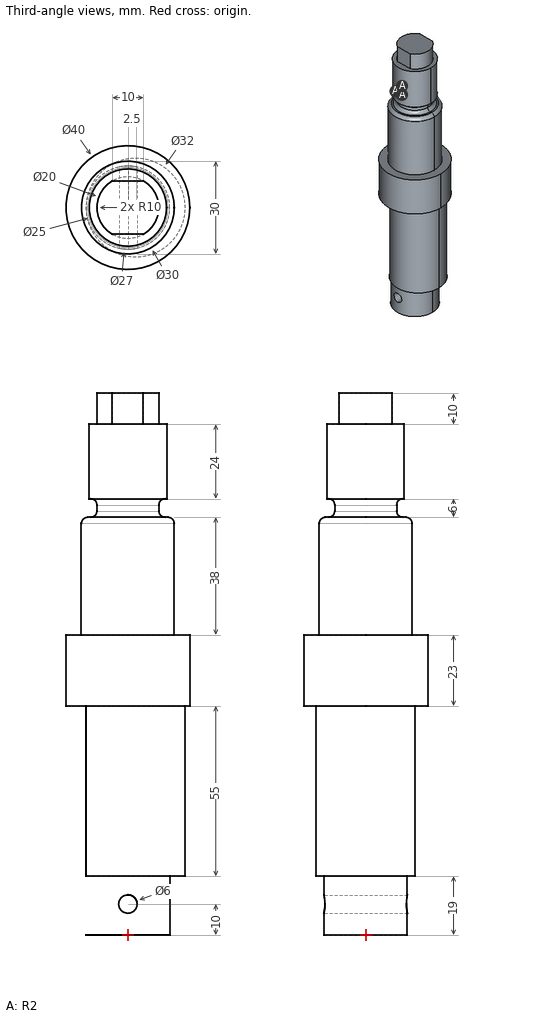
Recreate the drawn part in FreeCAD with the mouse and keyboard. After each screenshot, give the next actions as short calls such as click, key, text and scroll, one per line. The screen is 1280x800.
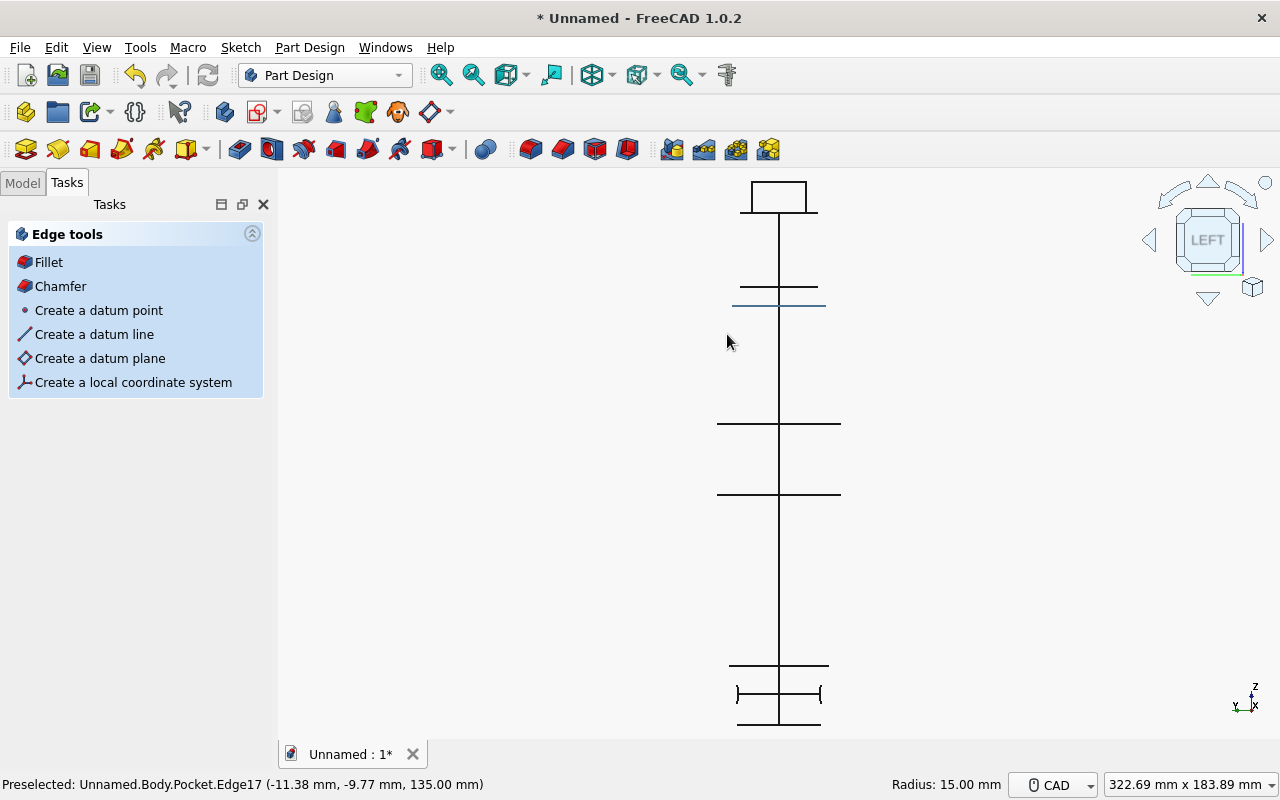
key(0)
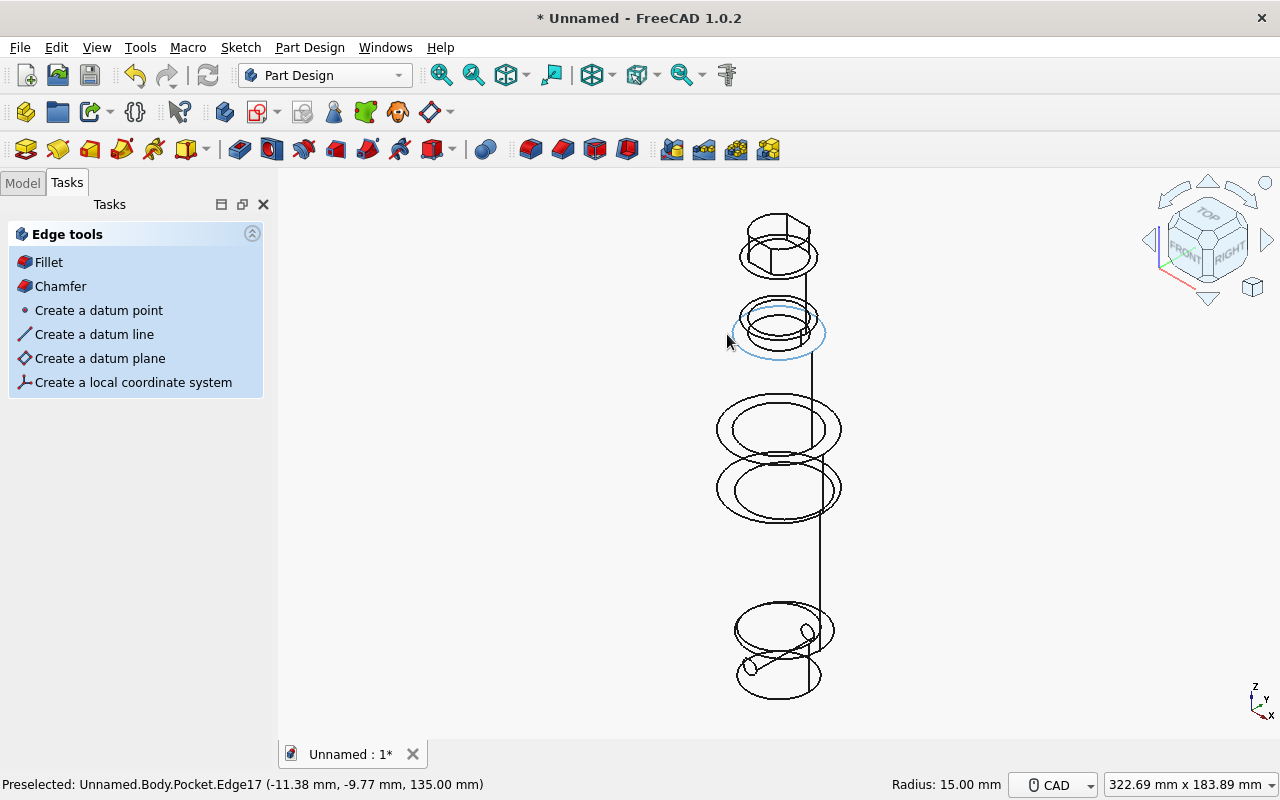
click(757, 319, ctrl)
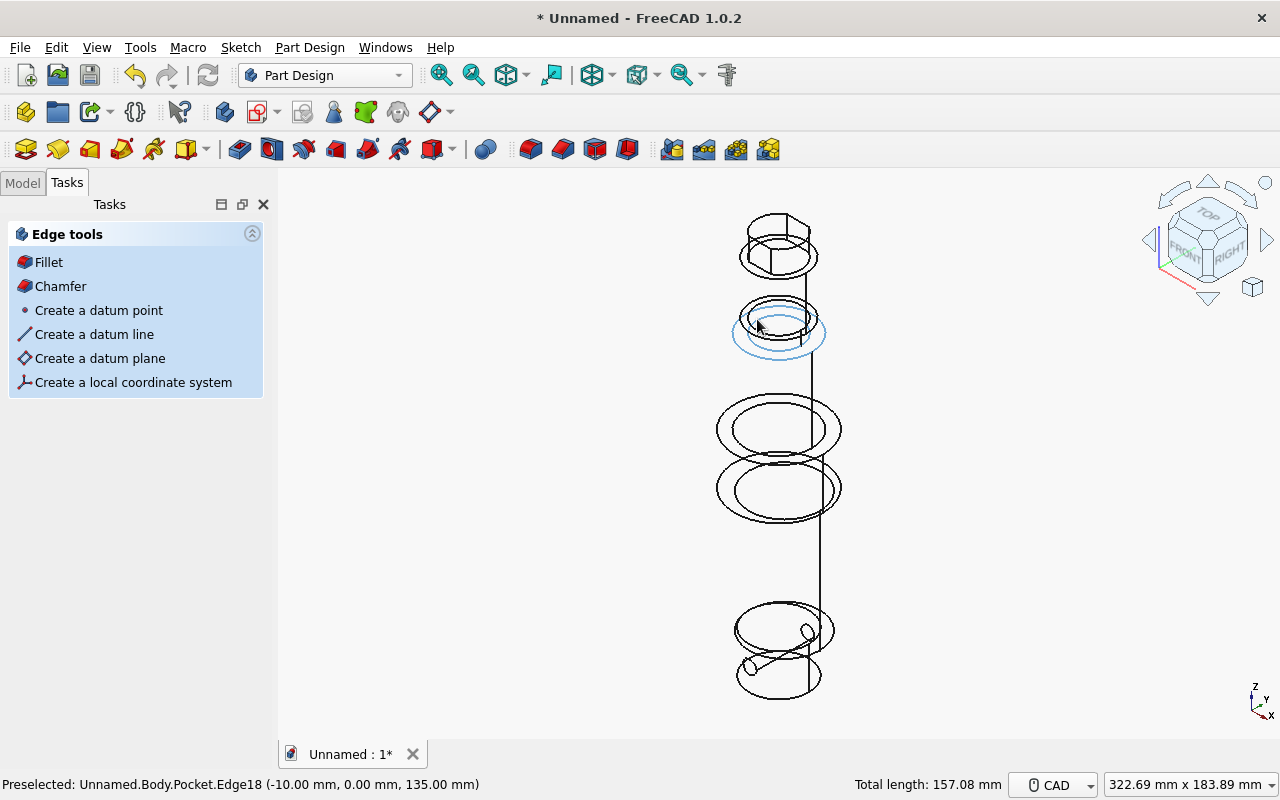
click(757, 304, ctrl)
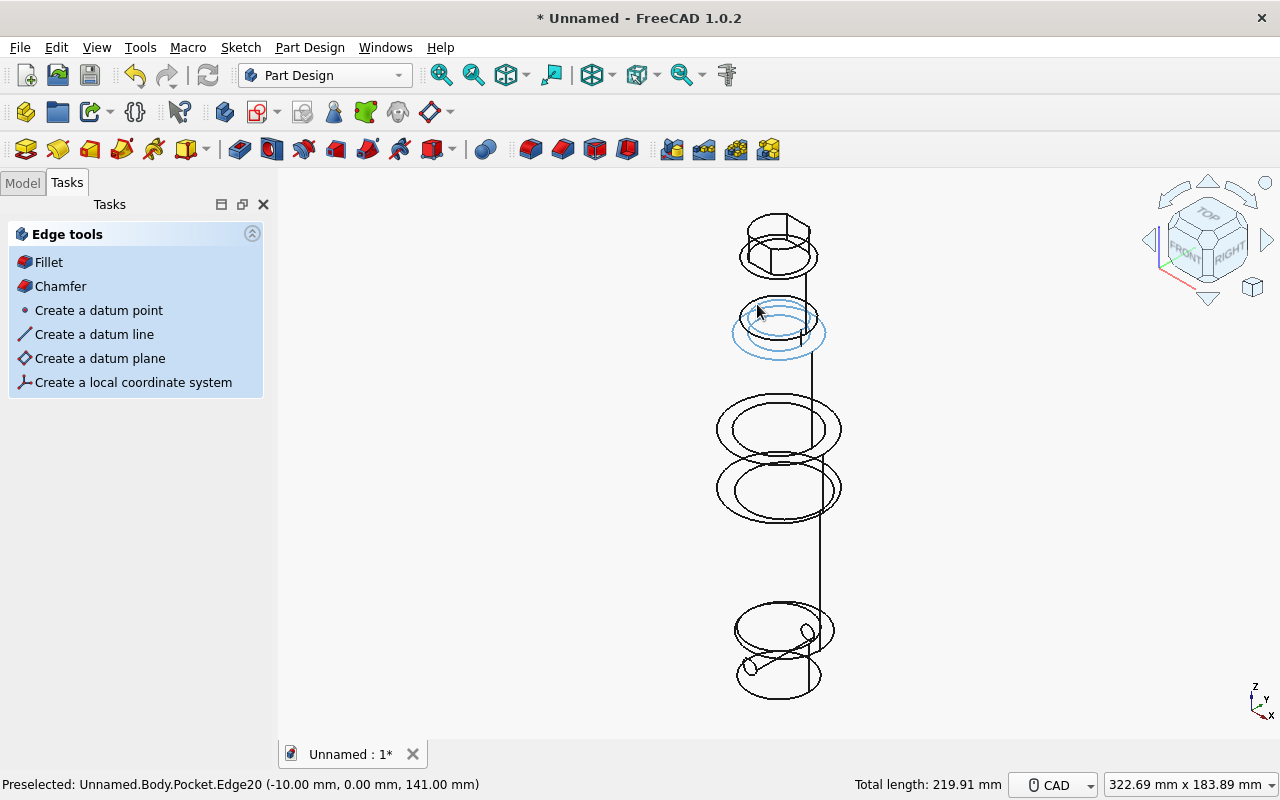
key(v)
key(1)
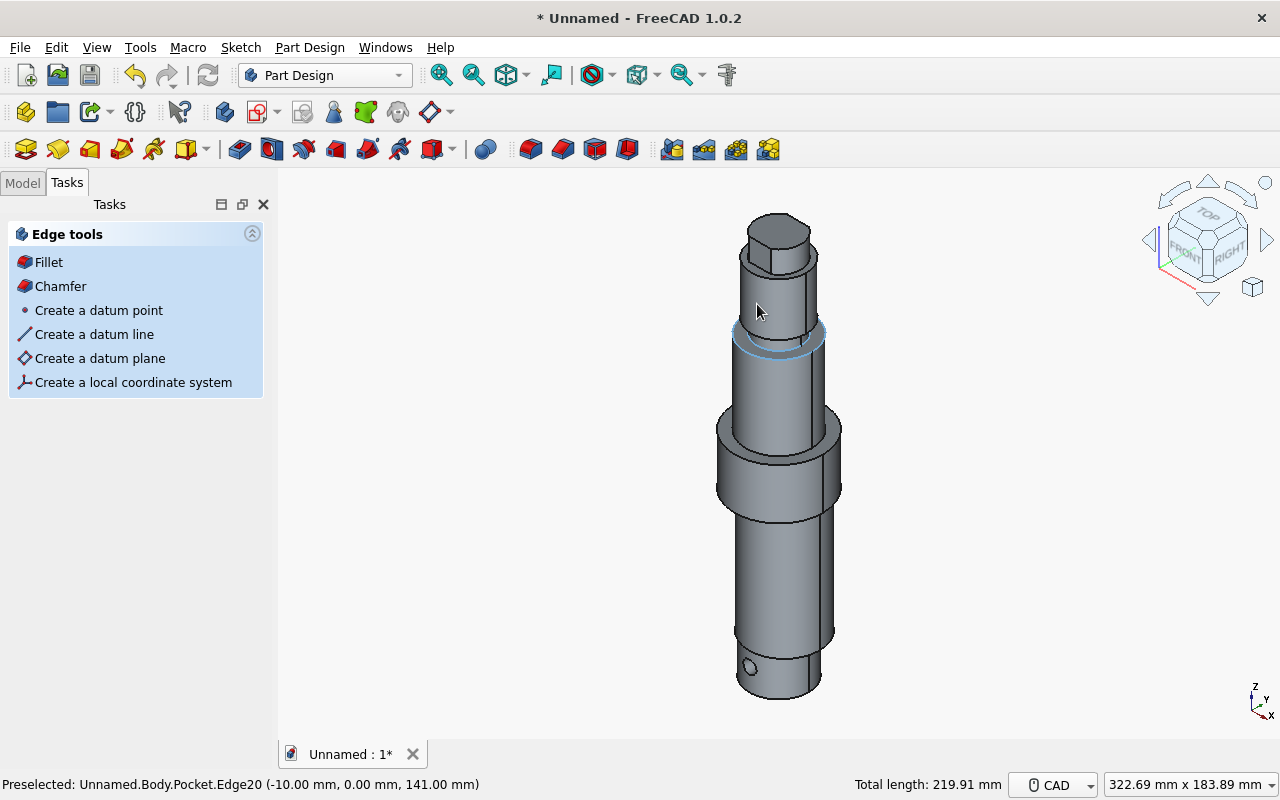
click(532, 150)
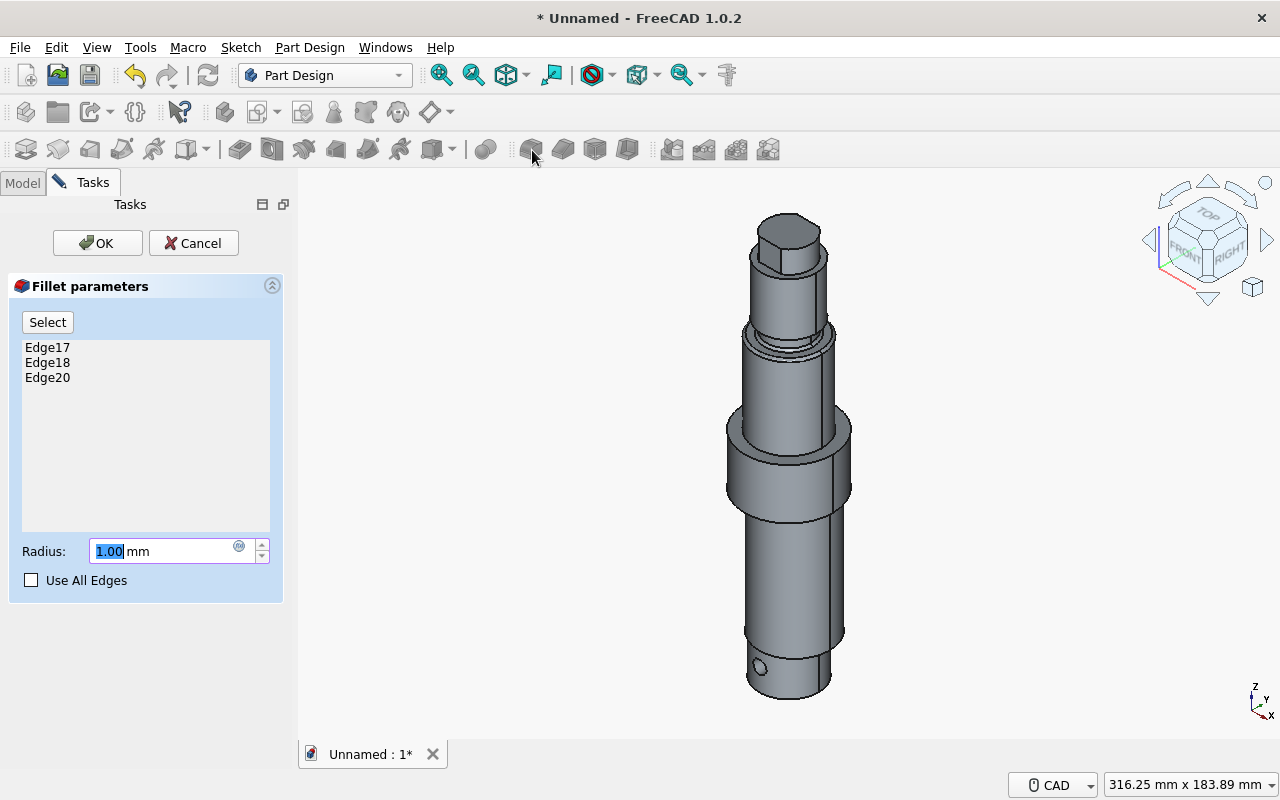
text(2)
key(Tab)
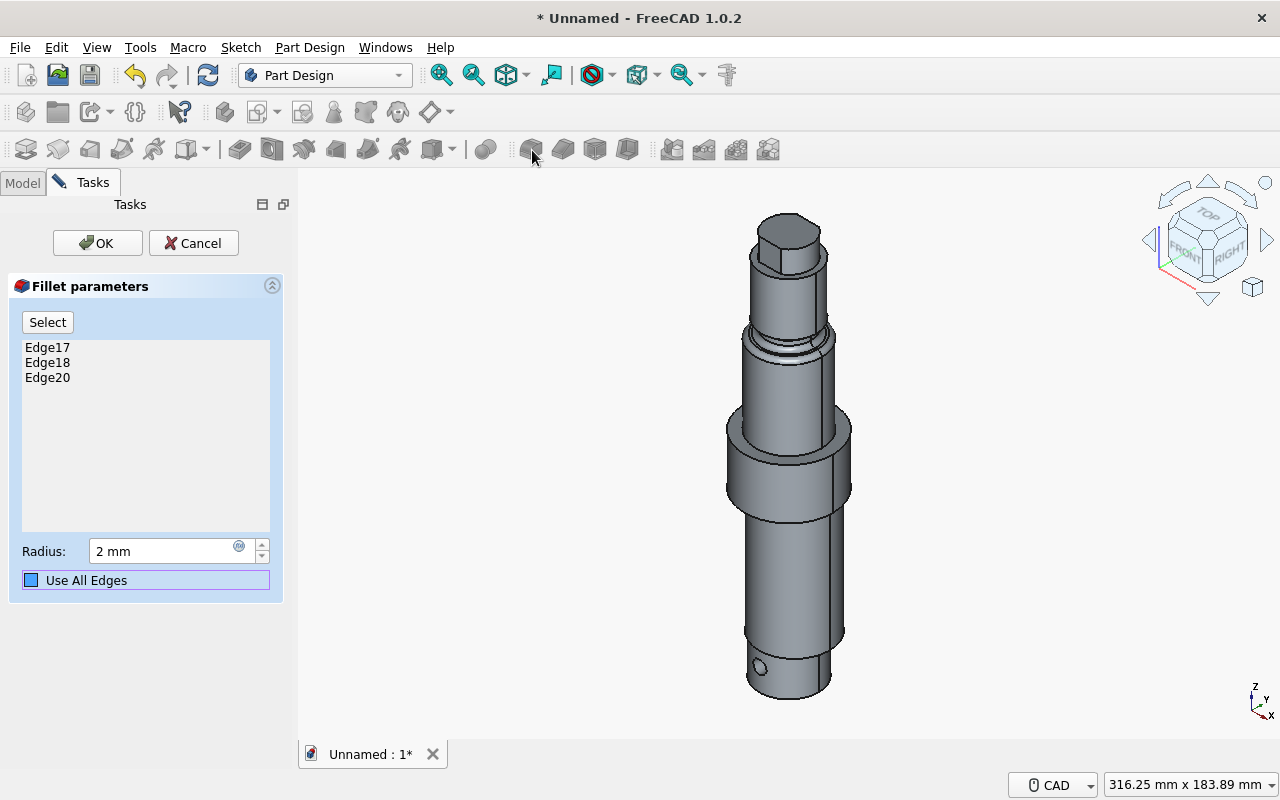
click(98, 243)